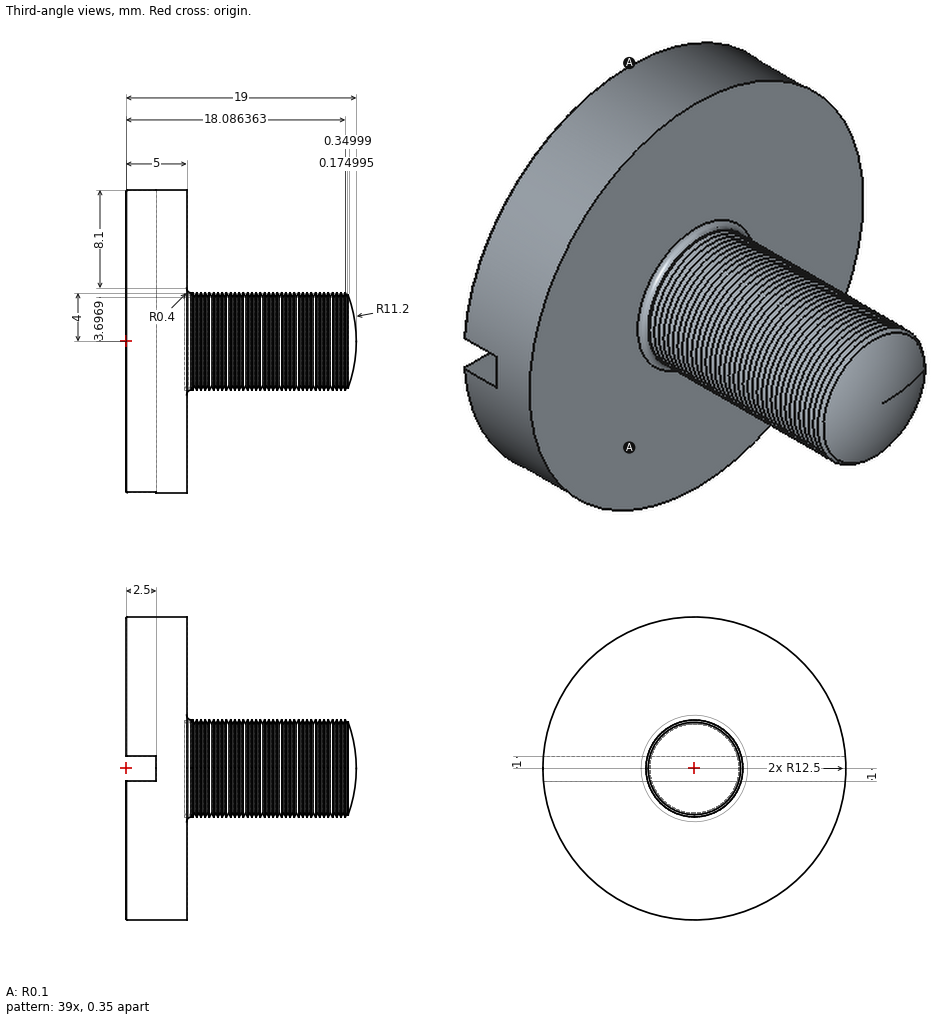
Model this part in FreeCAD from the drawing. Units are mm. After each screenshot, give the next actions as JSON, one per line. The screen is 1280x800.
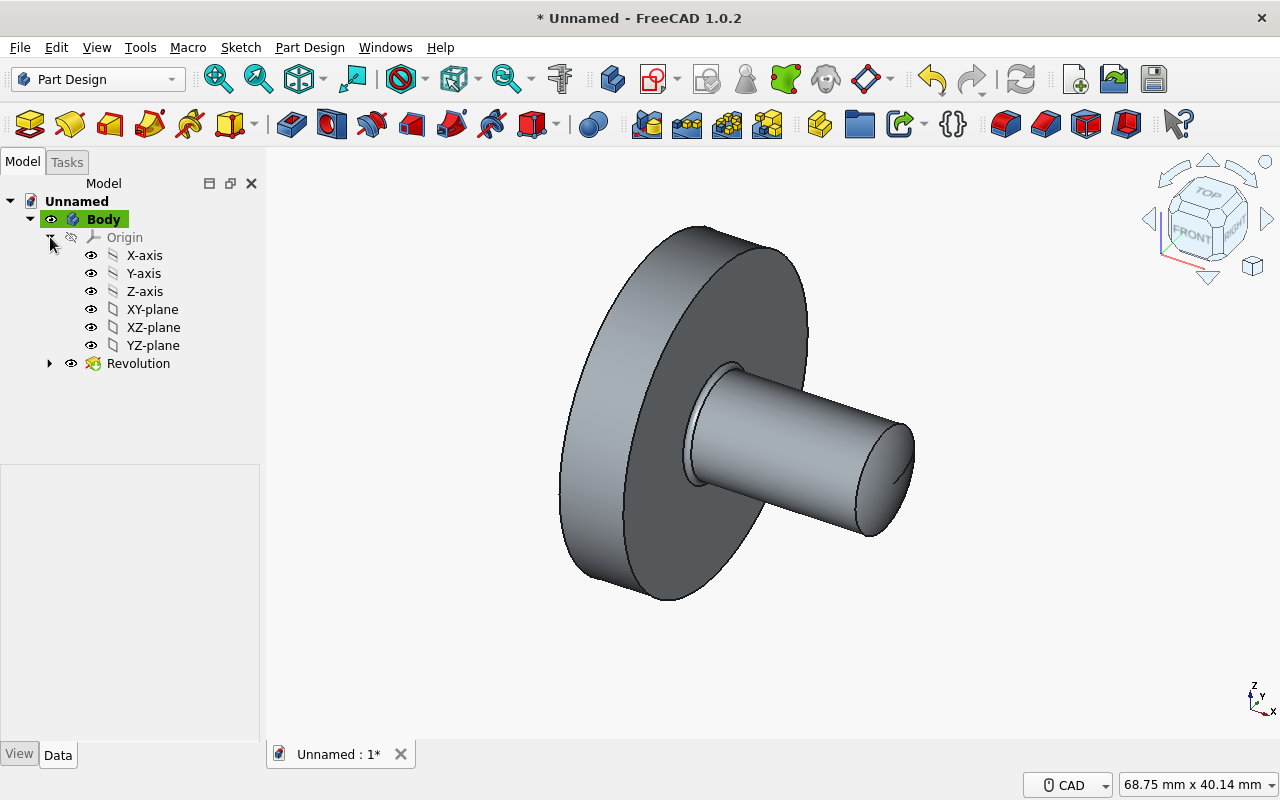
{"action": "left_click", "coordinate": [136, 345]}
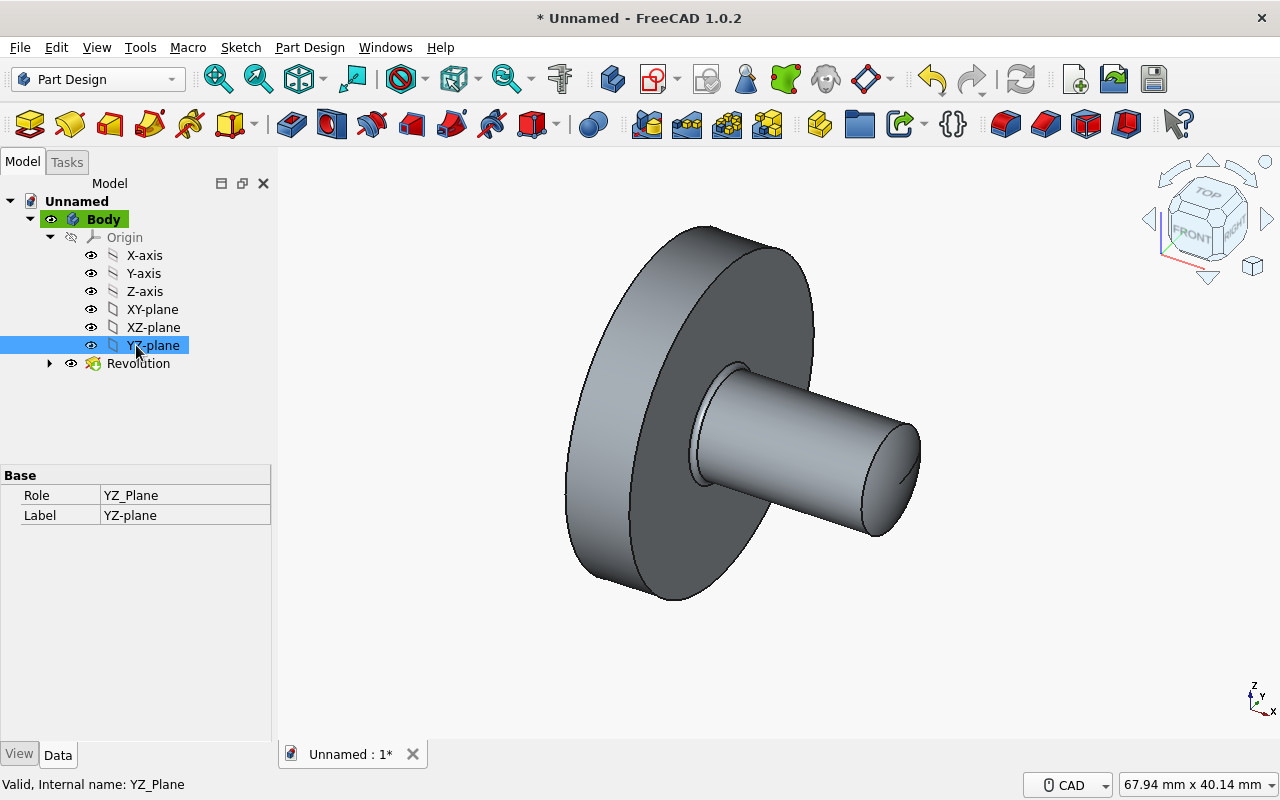
{"action": "left_click", "coordinate": [866, 80]}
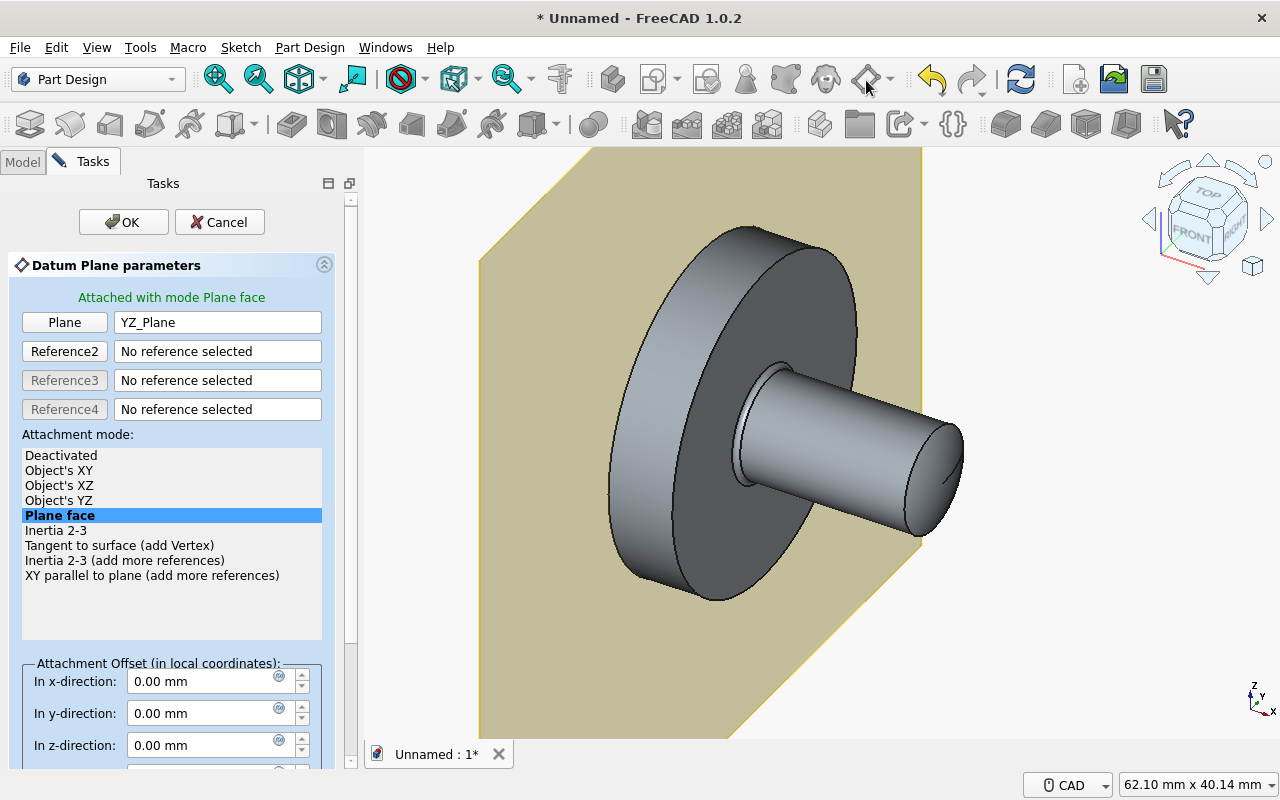
{"action": "triple_click", "coordinate": [210, 745]}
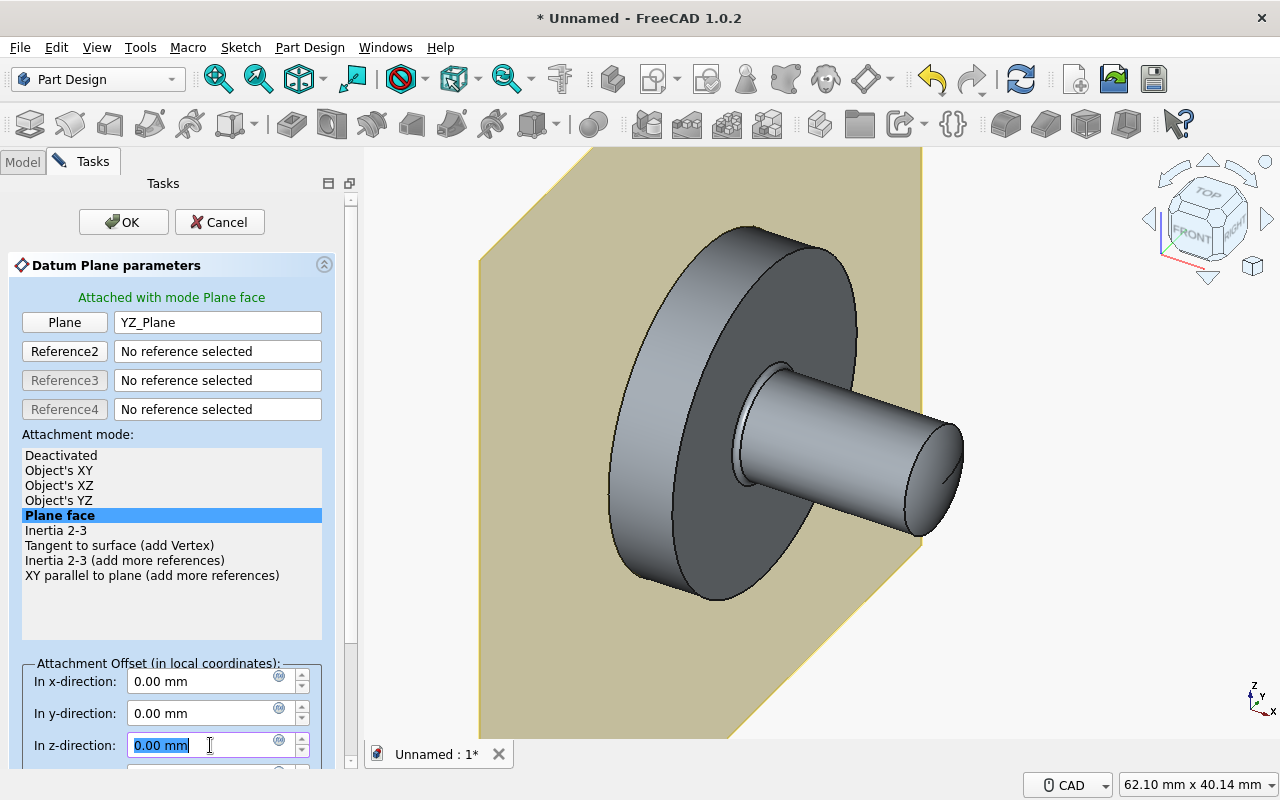
{"action": "type", "text": "2.5"}
{"action": "key", "text": "Tab"}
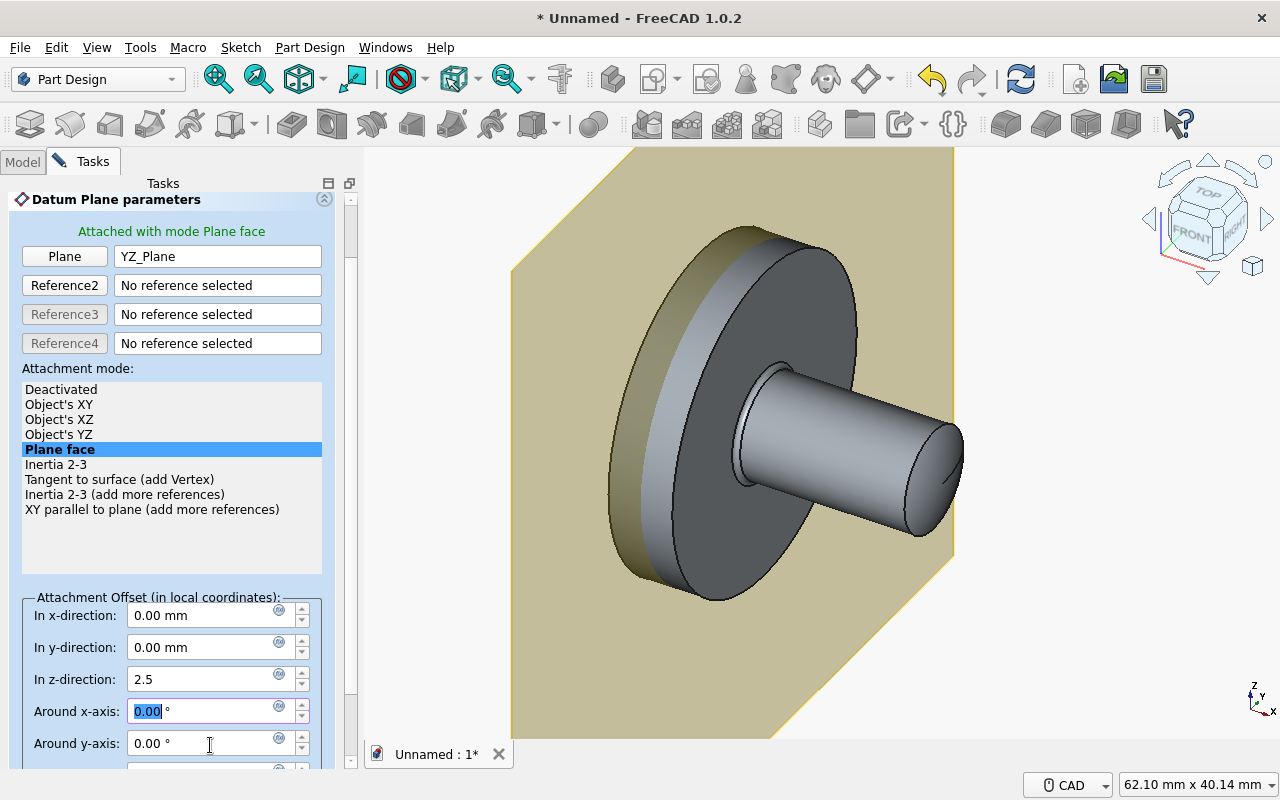
{"action": "scroll", "coordinate": [351, 480], "scroll_direction": "up", "scroll_amount": 2}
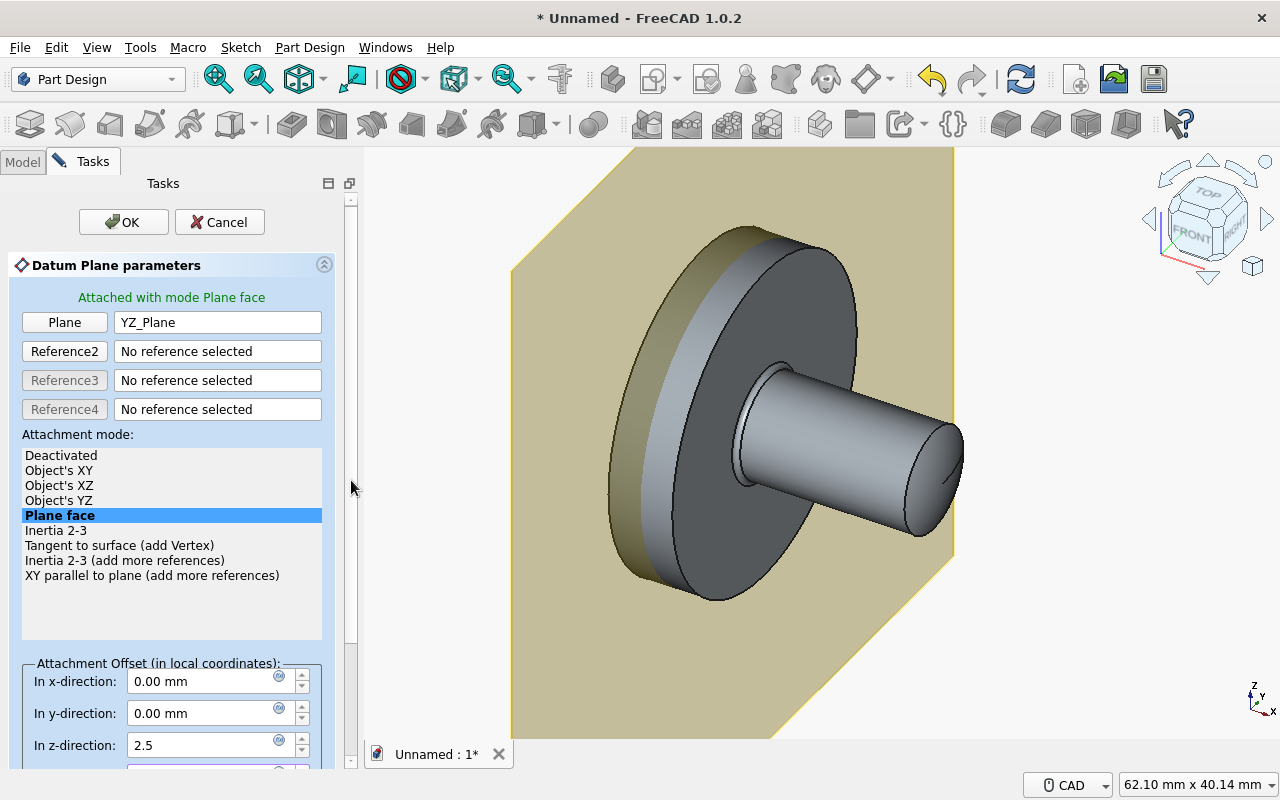
{"action": "left_click", "coordinate": [124, 222]}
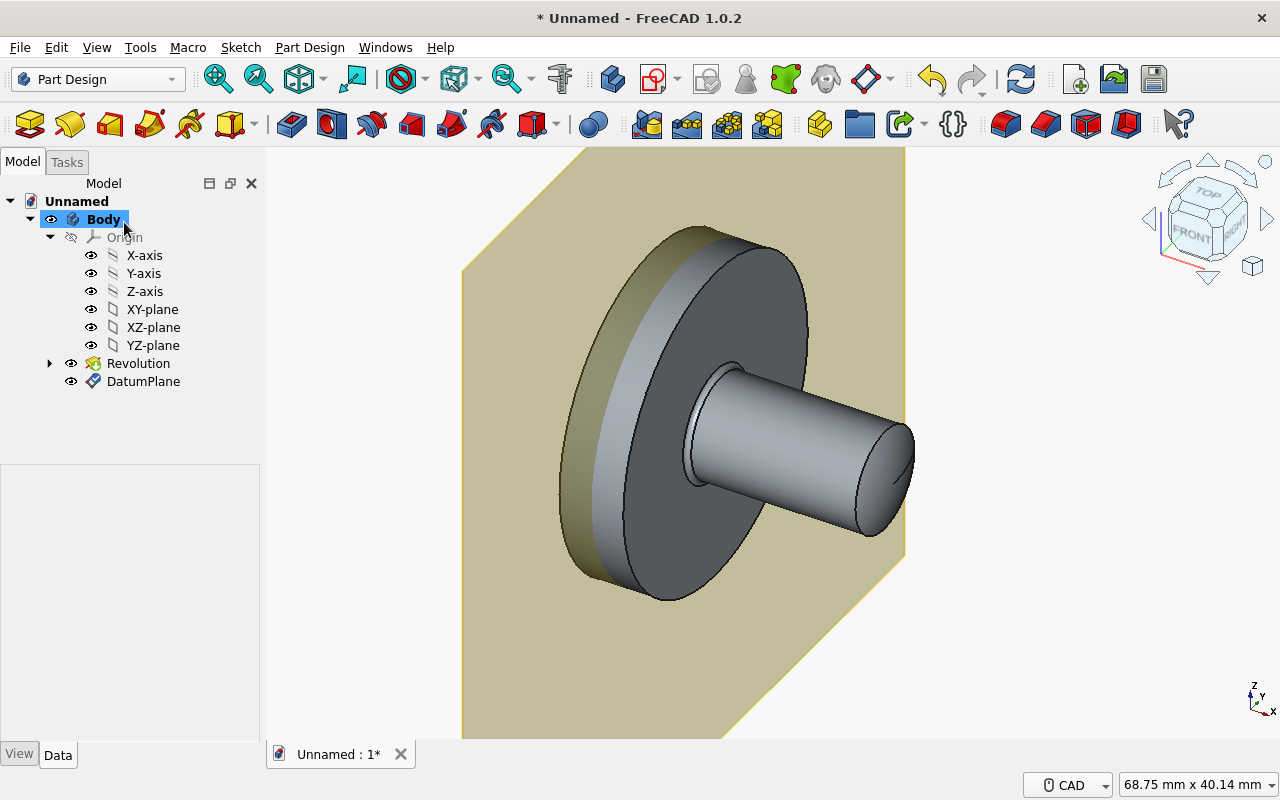
{"action": "left_click", "coordinate": [116, 381]}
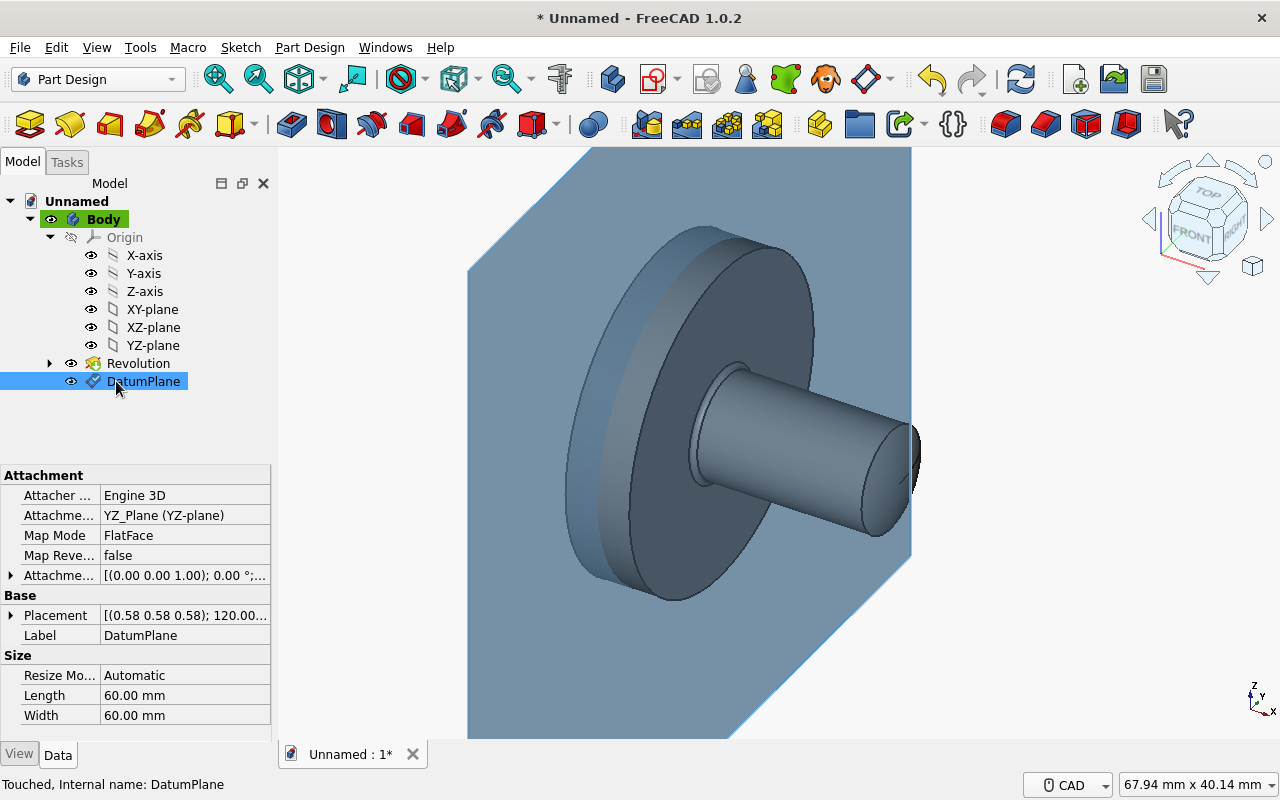
{"action": "left_click", "coordinate": [654, 80]}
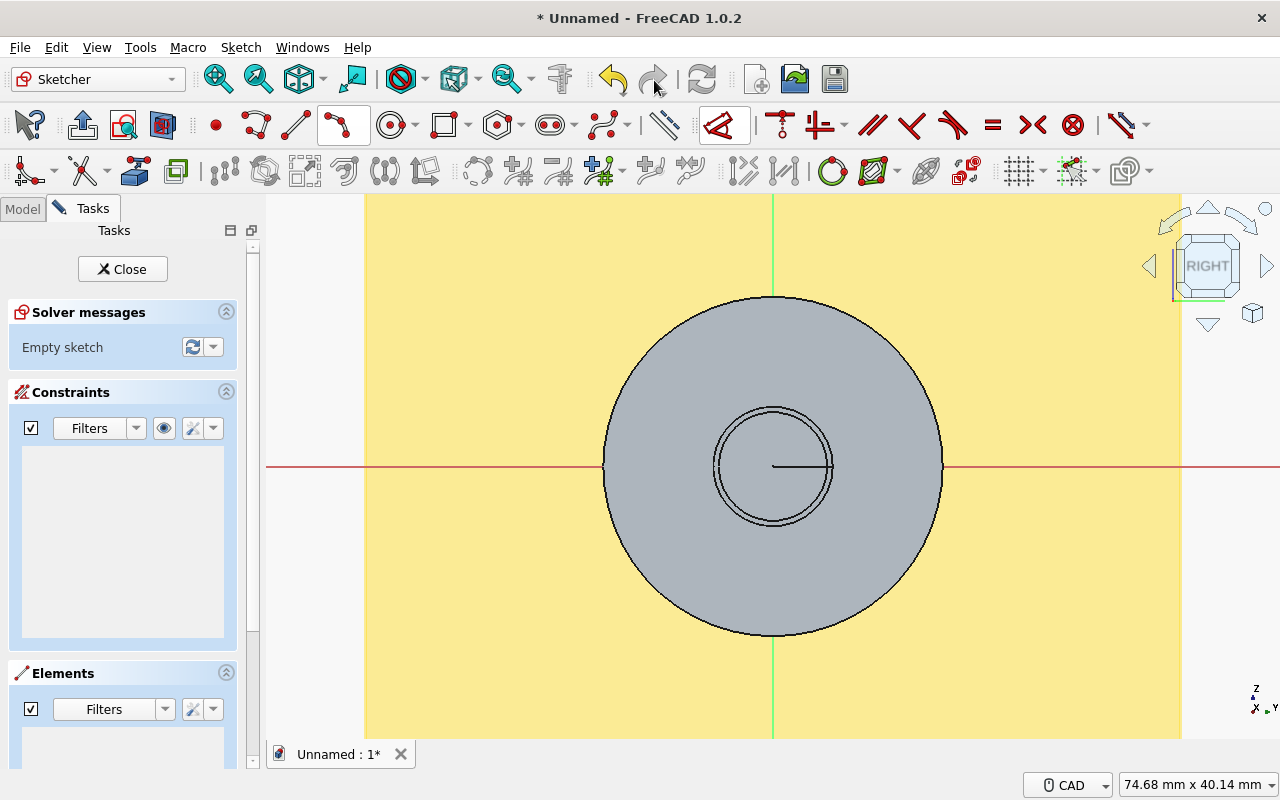
{"action": "left_click", "coordinate": [164, 126]}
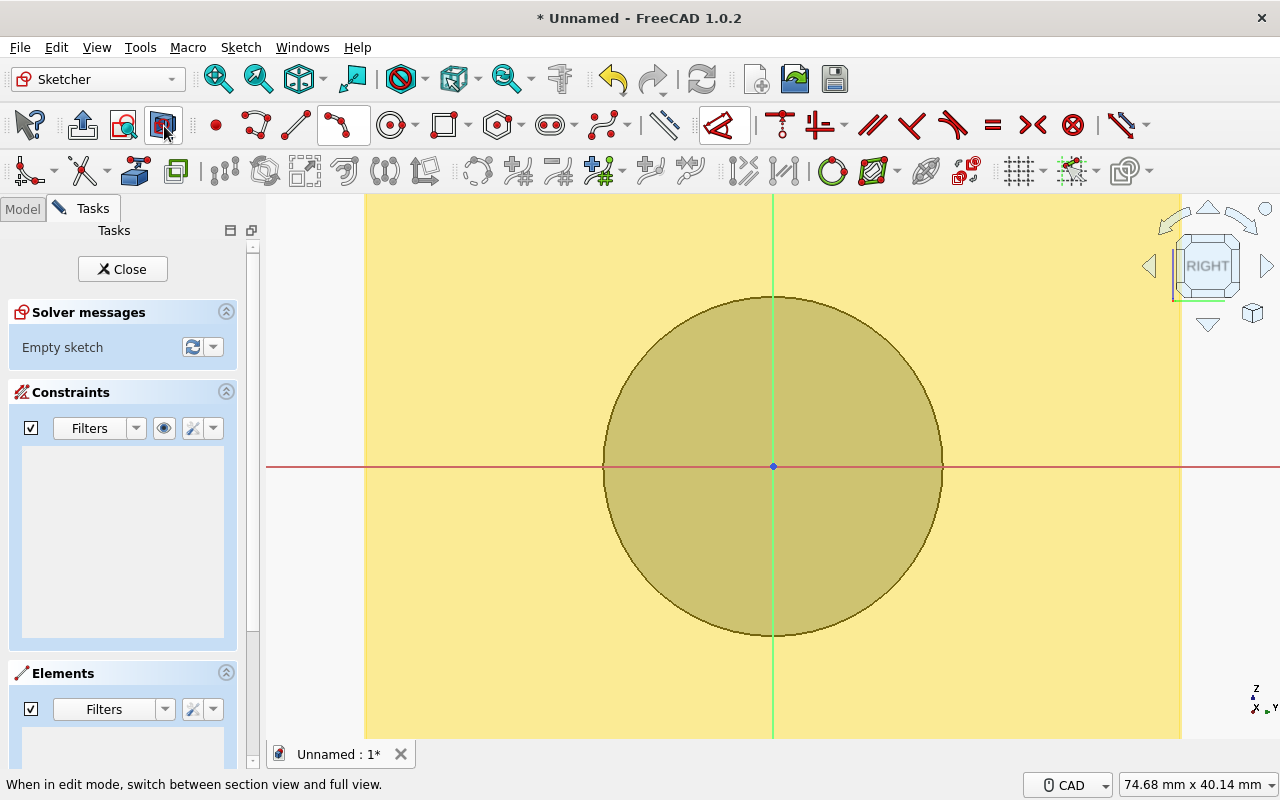
{"action": "scroll", "coordinate": [856, 466], "scroll_direction": "up", "scroll_amount": 3}